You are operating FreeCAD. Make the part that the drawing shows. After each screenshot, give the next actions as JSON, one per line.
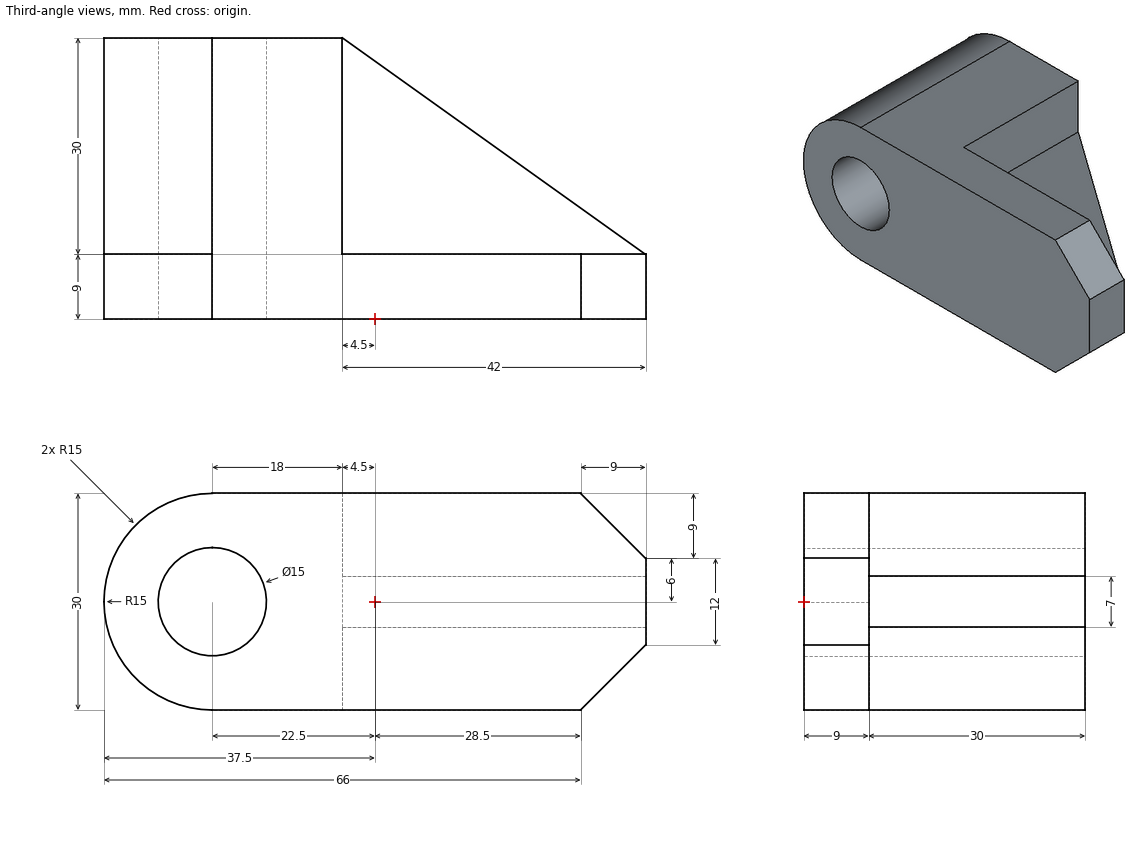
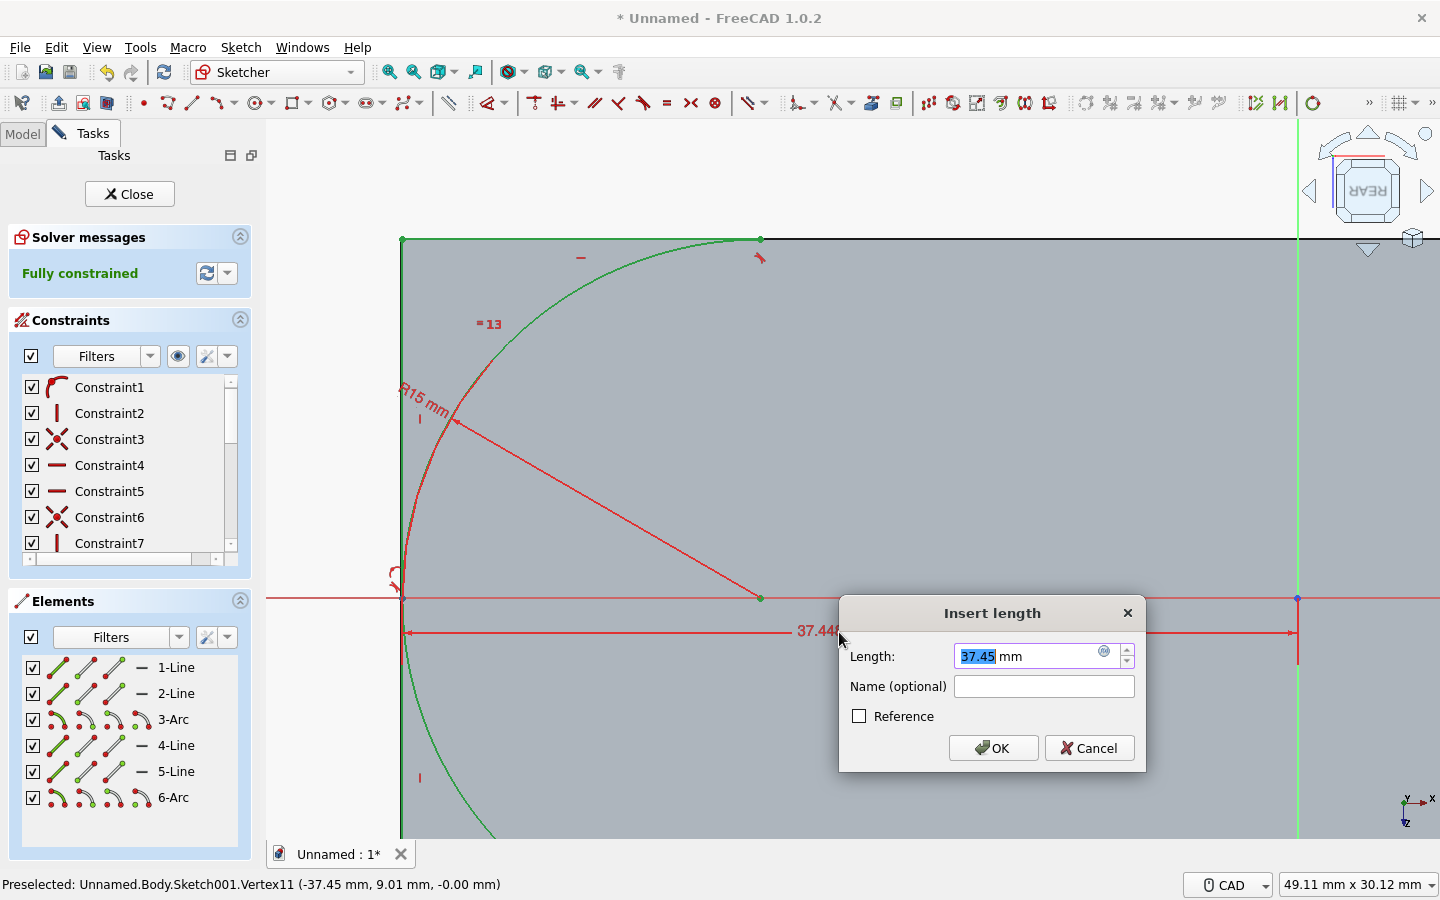
{"action": "type", "text": "37.5"}
{"action": "key", "text": "Return"}
{"action": "key", "text": "Escape"}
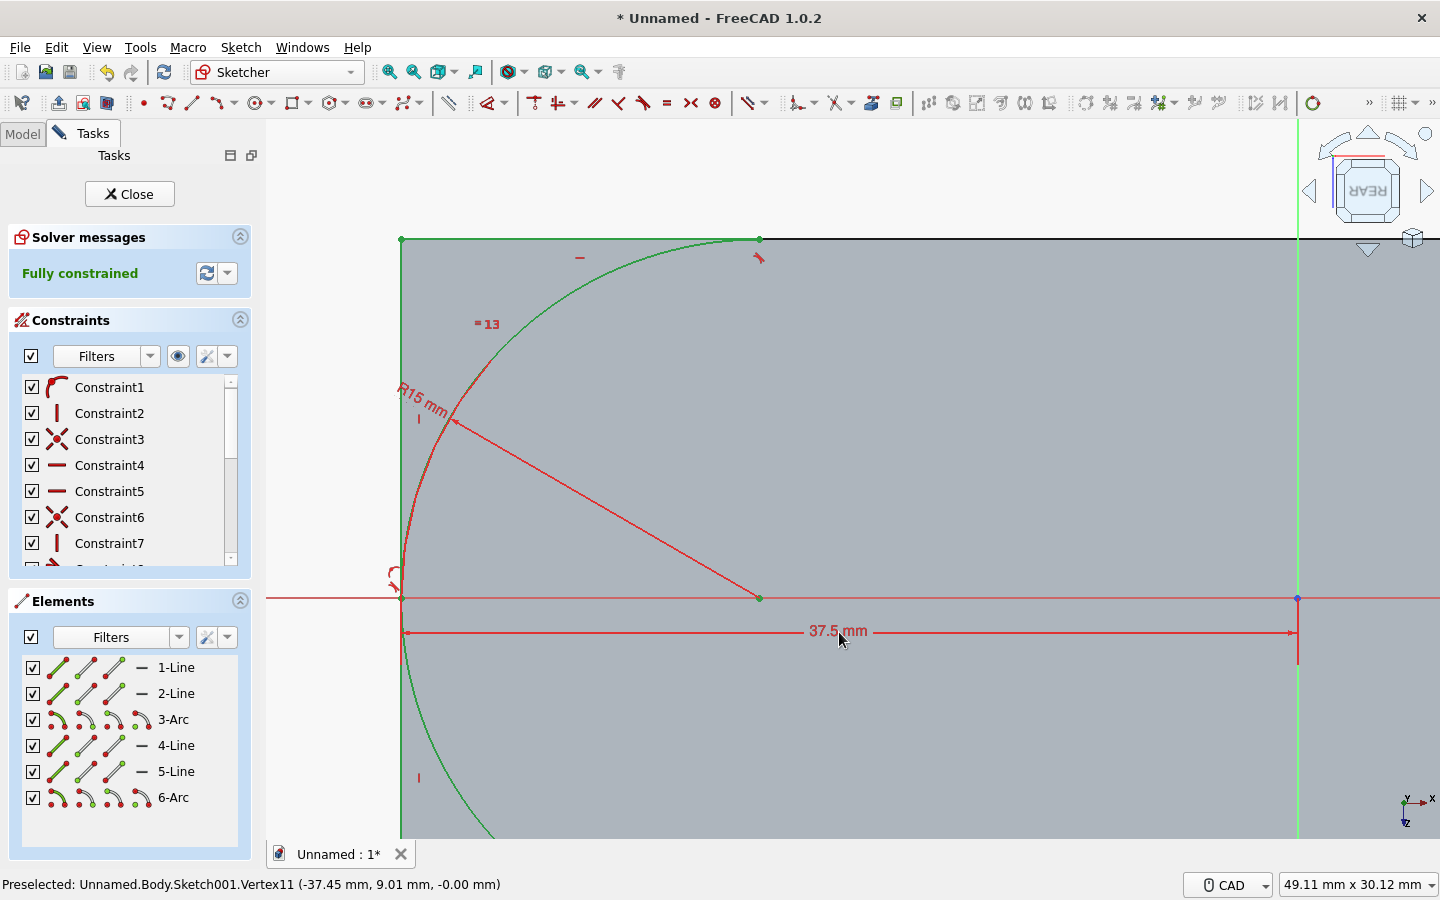
{"action": "left_click", "coordinate": [130, 194]}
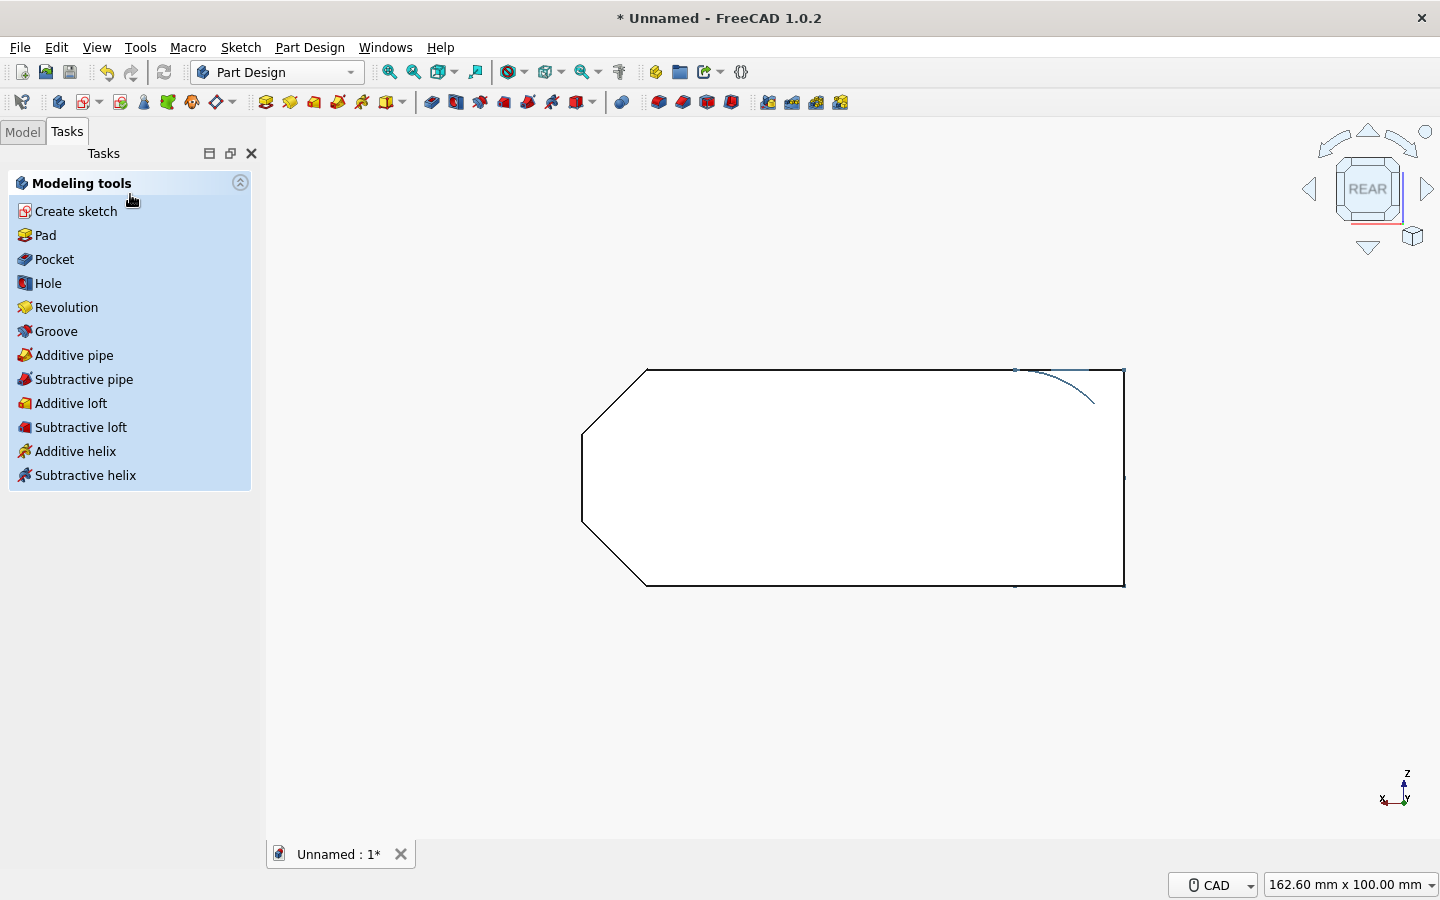
{"action": "left_click", "coordinate": [432, 102]}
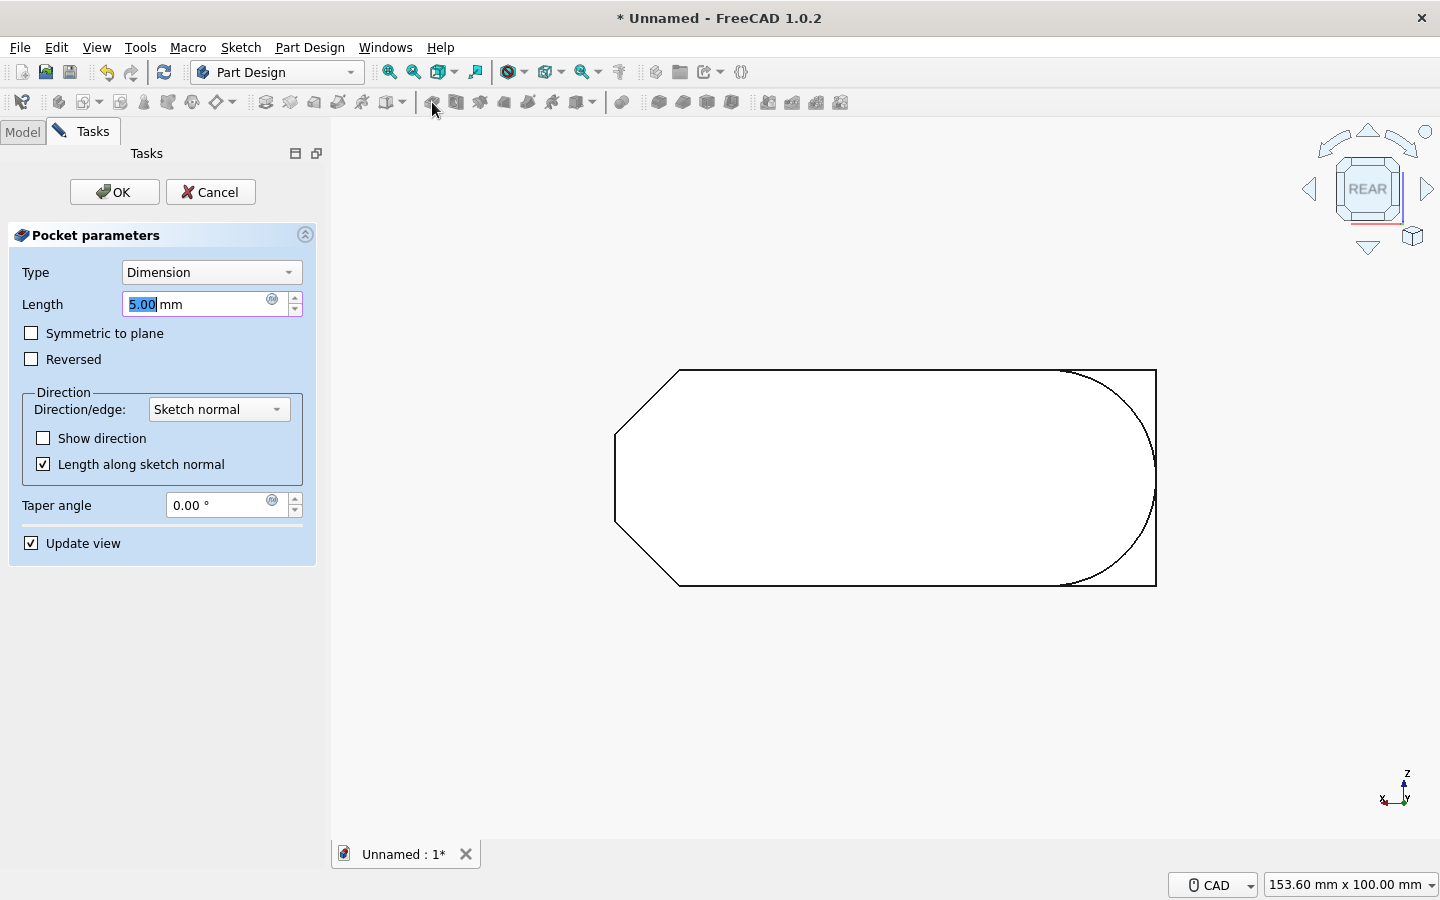
{"action": "type", "text": "9"}
{"action": "key", "text": "Tab"}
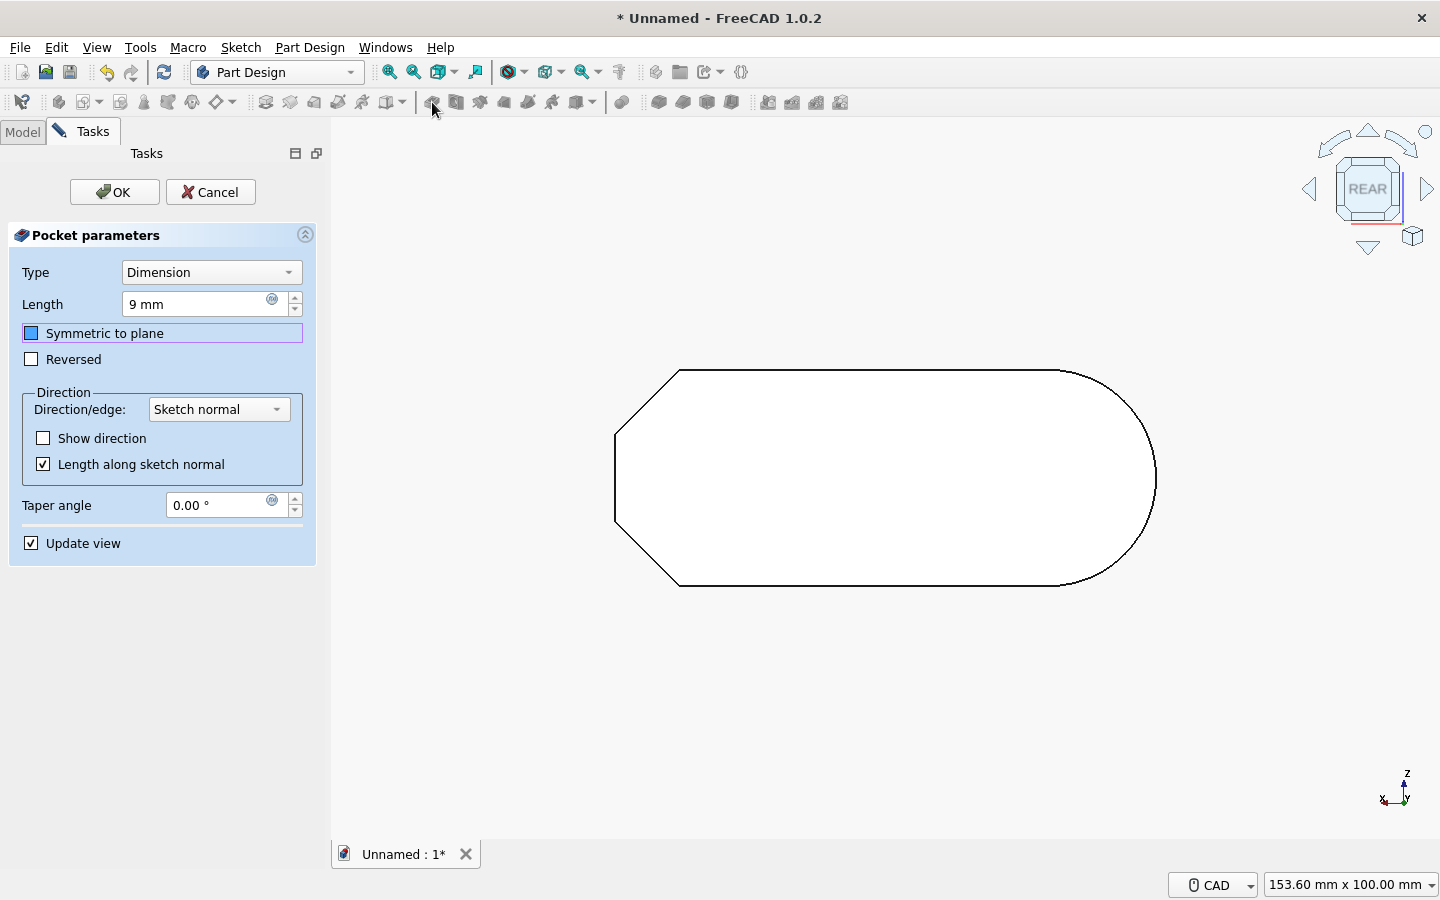
{"action": "left_click", "coordinate": [115, 192]}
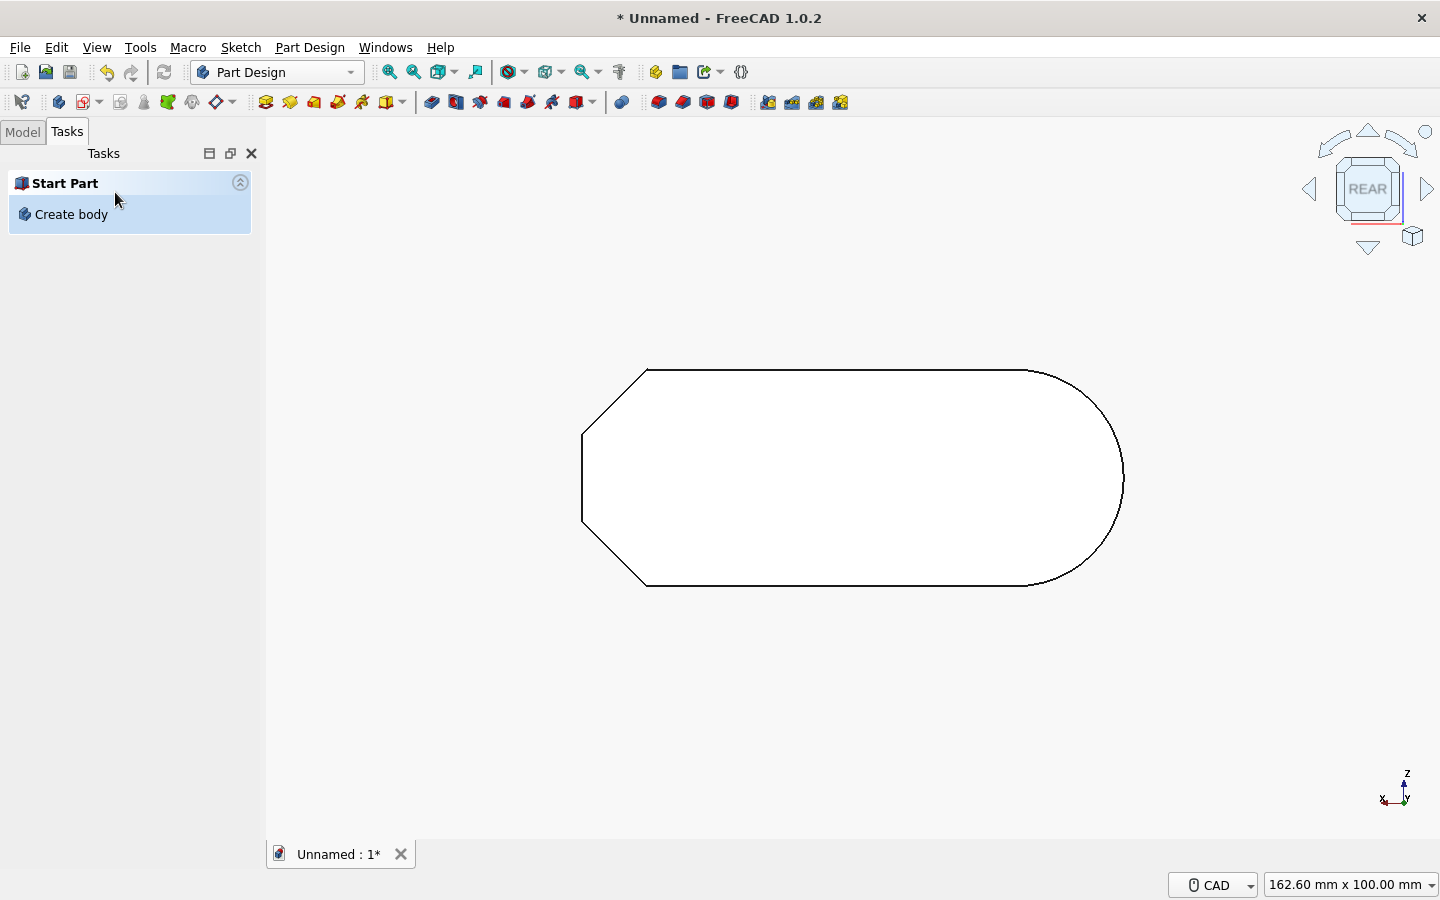
{"action": "left_click", "coordinate": [23, 131]}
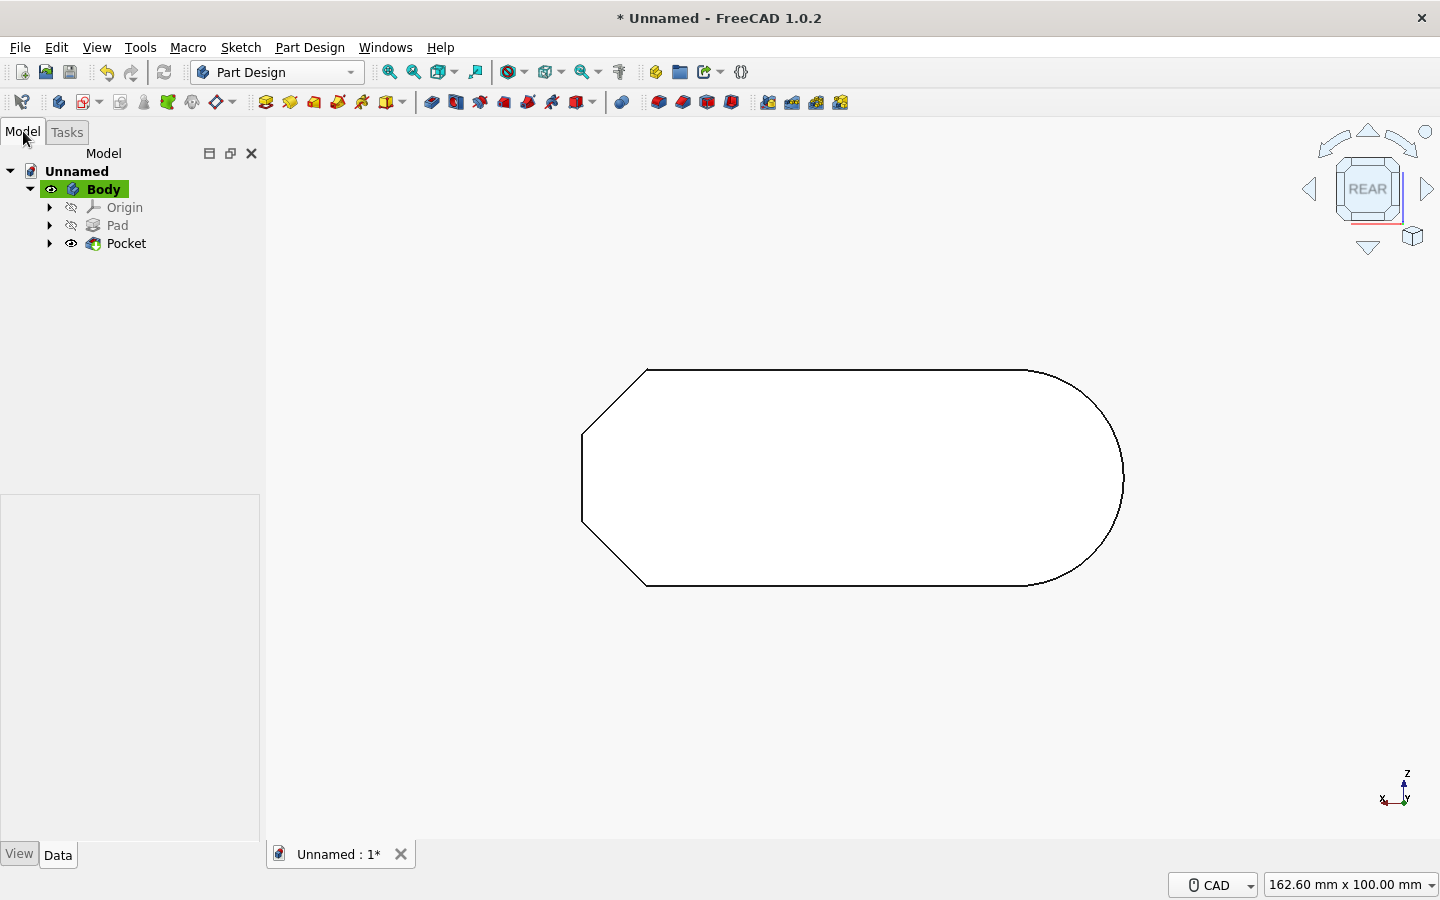
{"action": "left_click", "coordinate": [50, 207]}